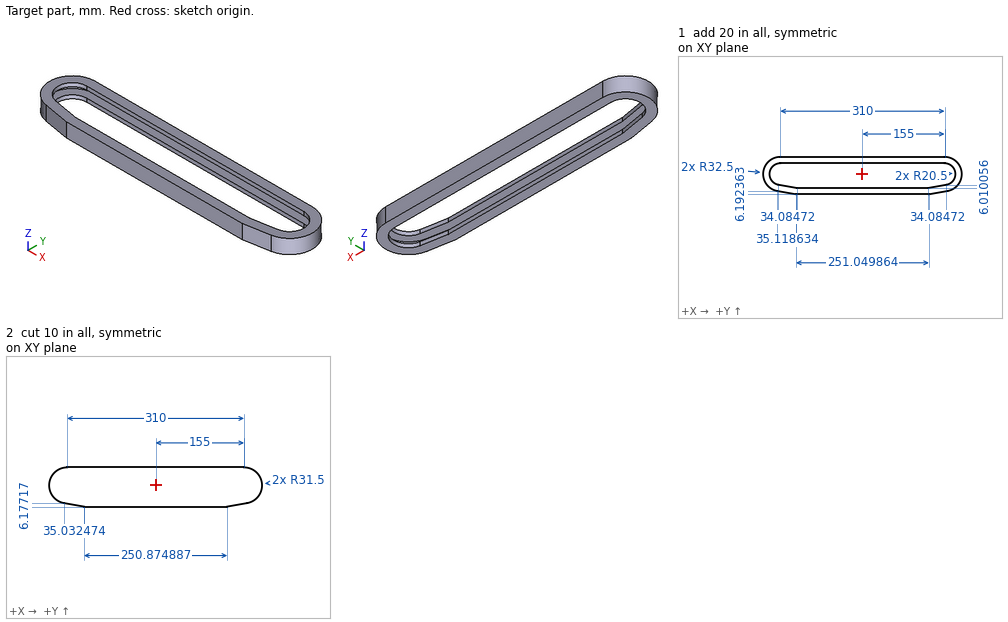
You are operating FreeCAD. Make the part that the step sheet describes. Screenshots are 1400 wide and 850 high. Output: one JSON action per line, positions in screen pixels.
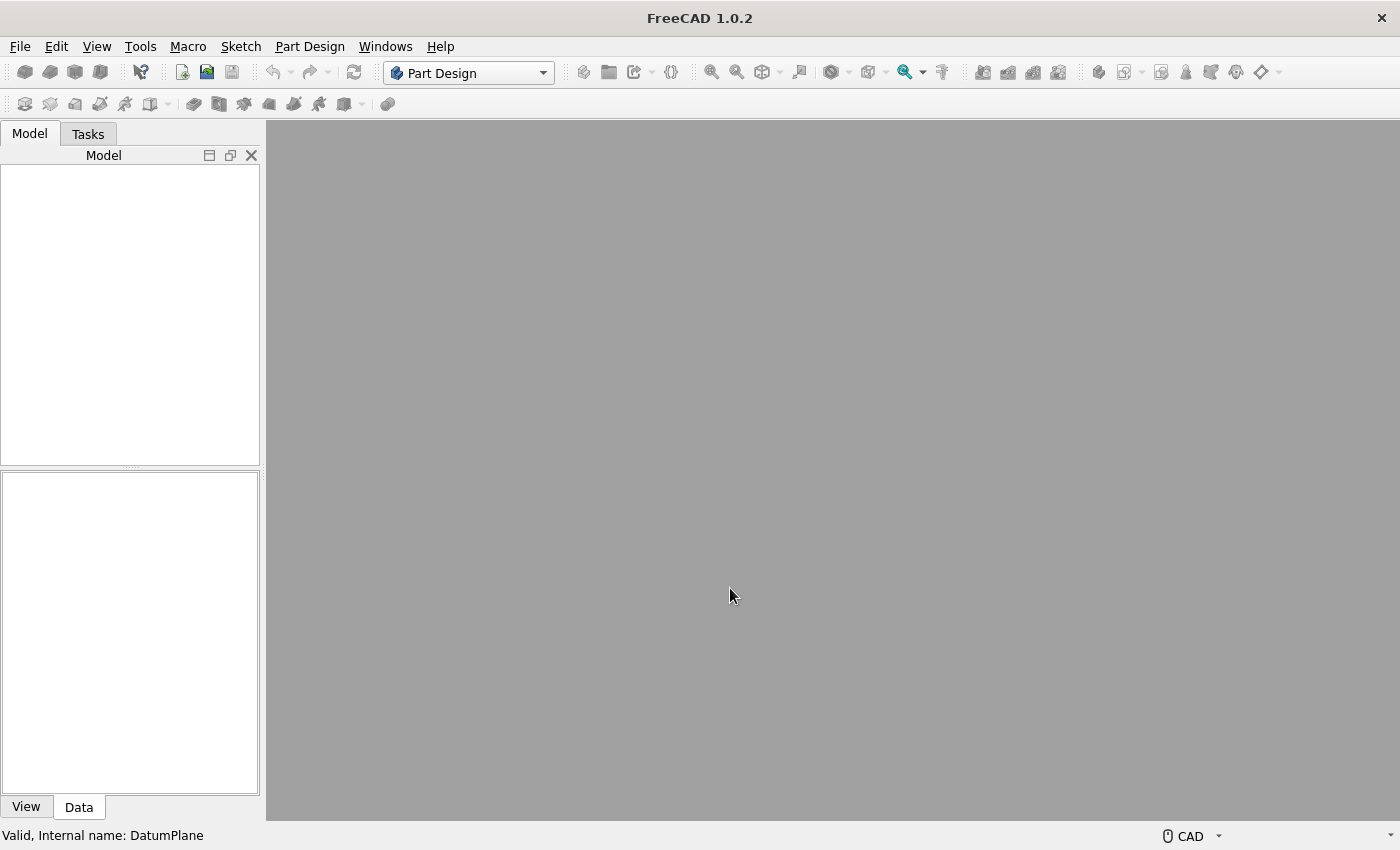
{"action": "left_click", "coordinate": [182, 72]}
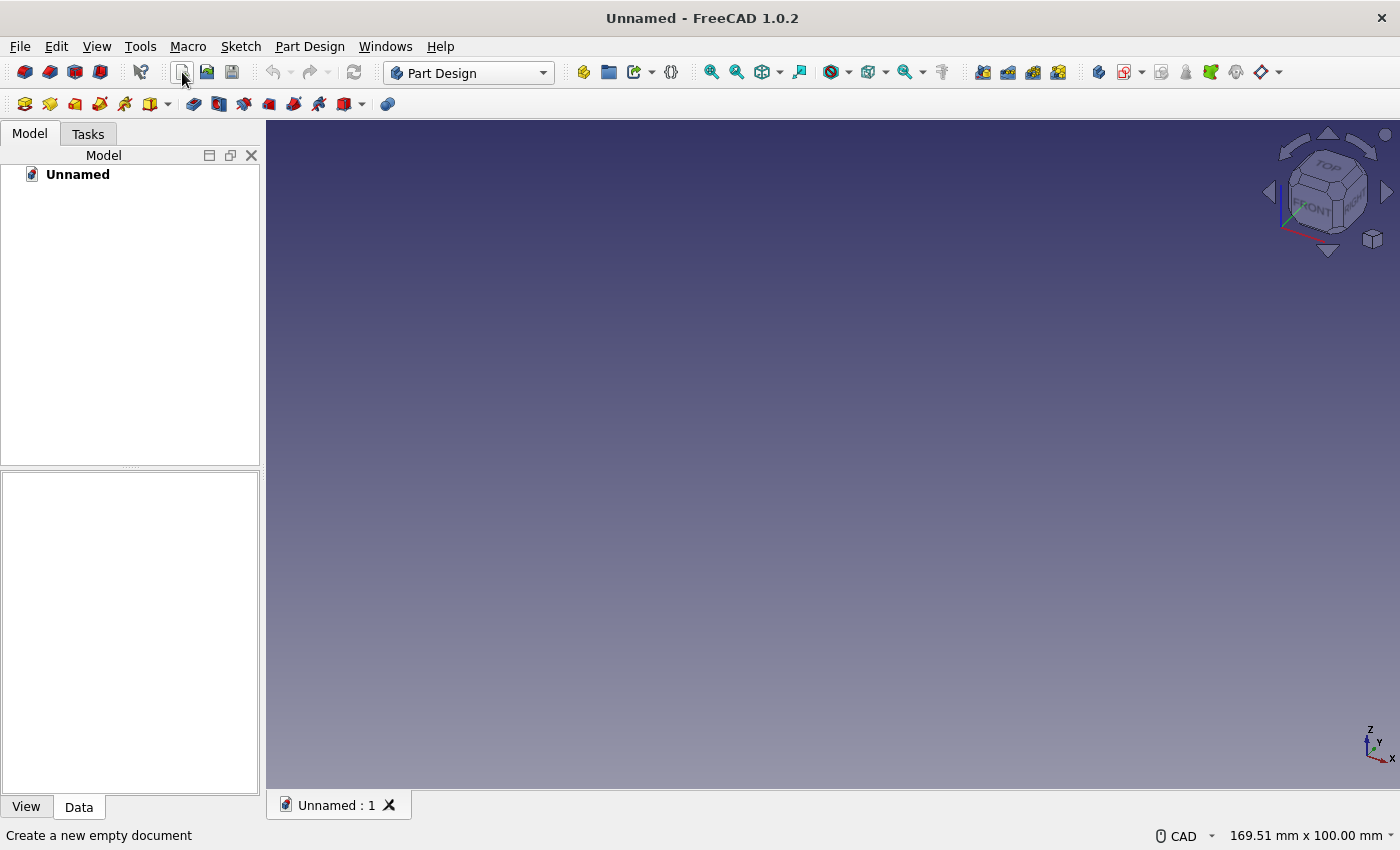
{"action": "left_click", "coordinate": [1124, 72]}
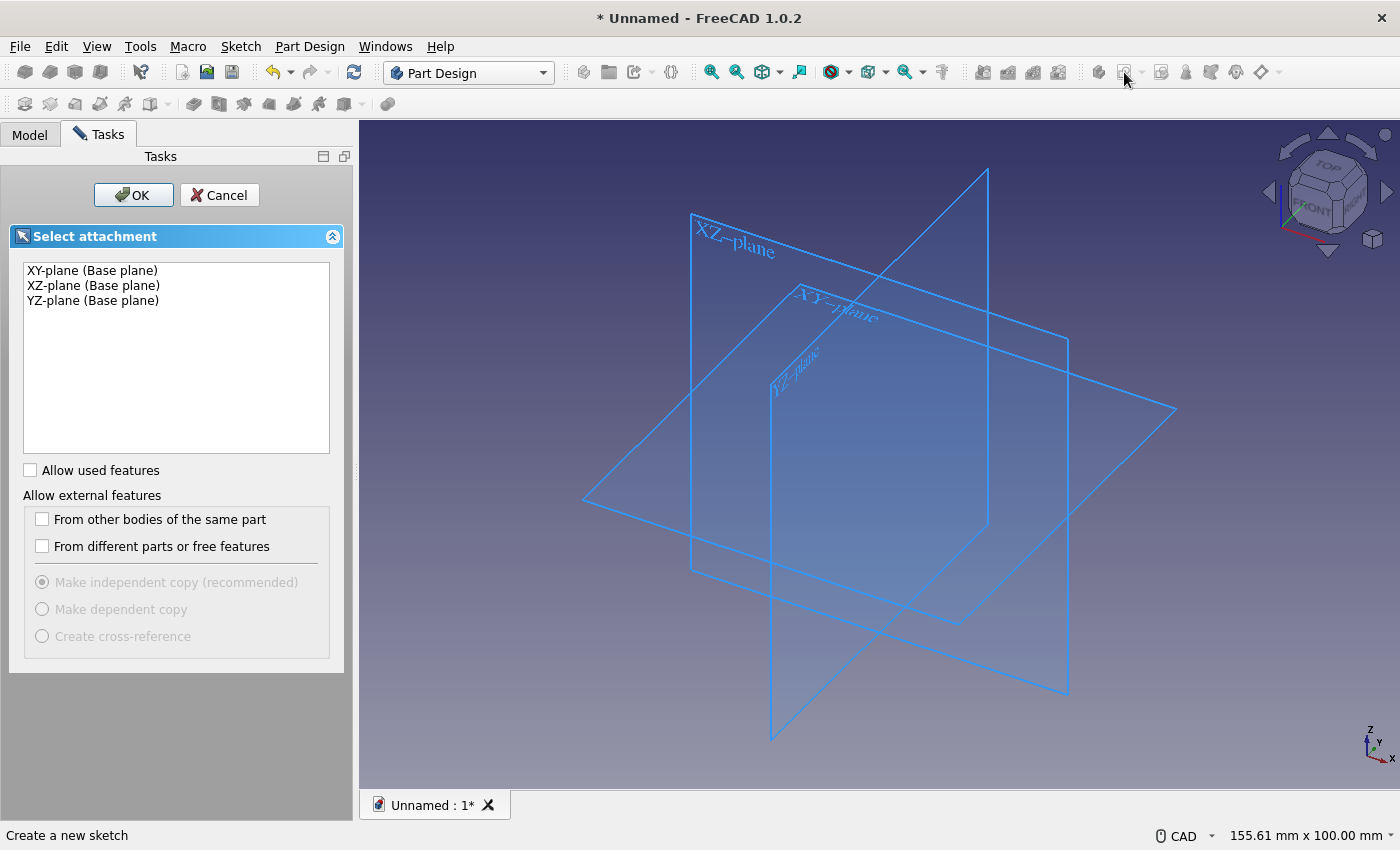
{"action": "left_click", "coordinate": [84, 270]}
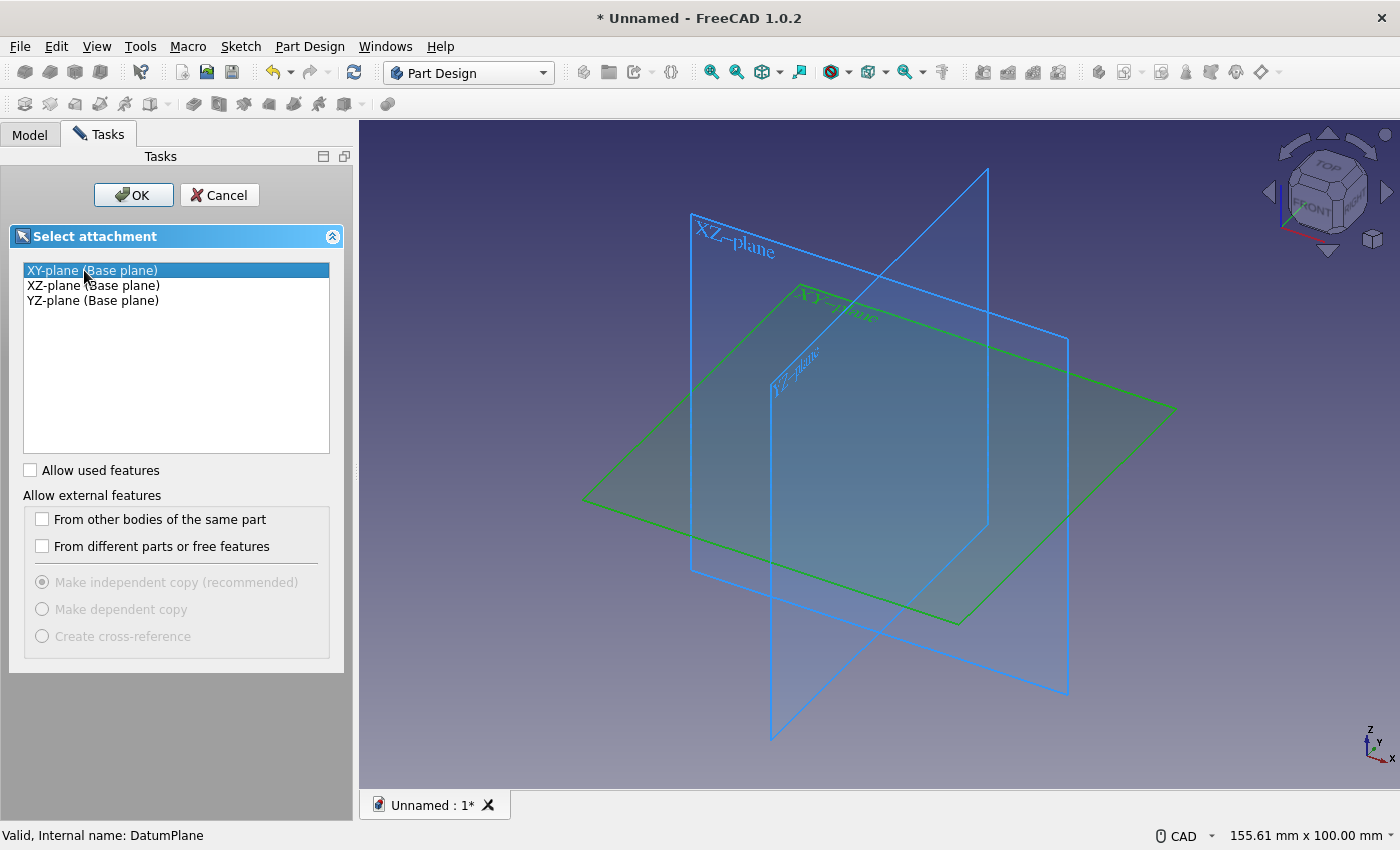
{"action": "left_click", "coordinate": [134, 195]}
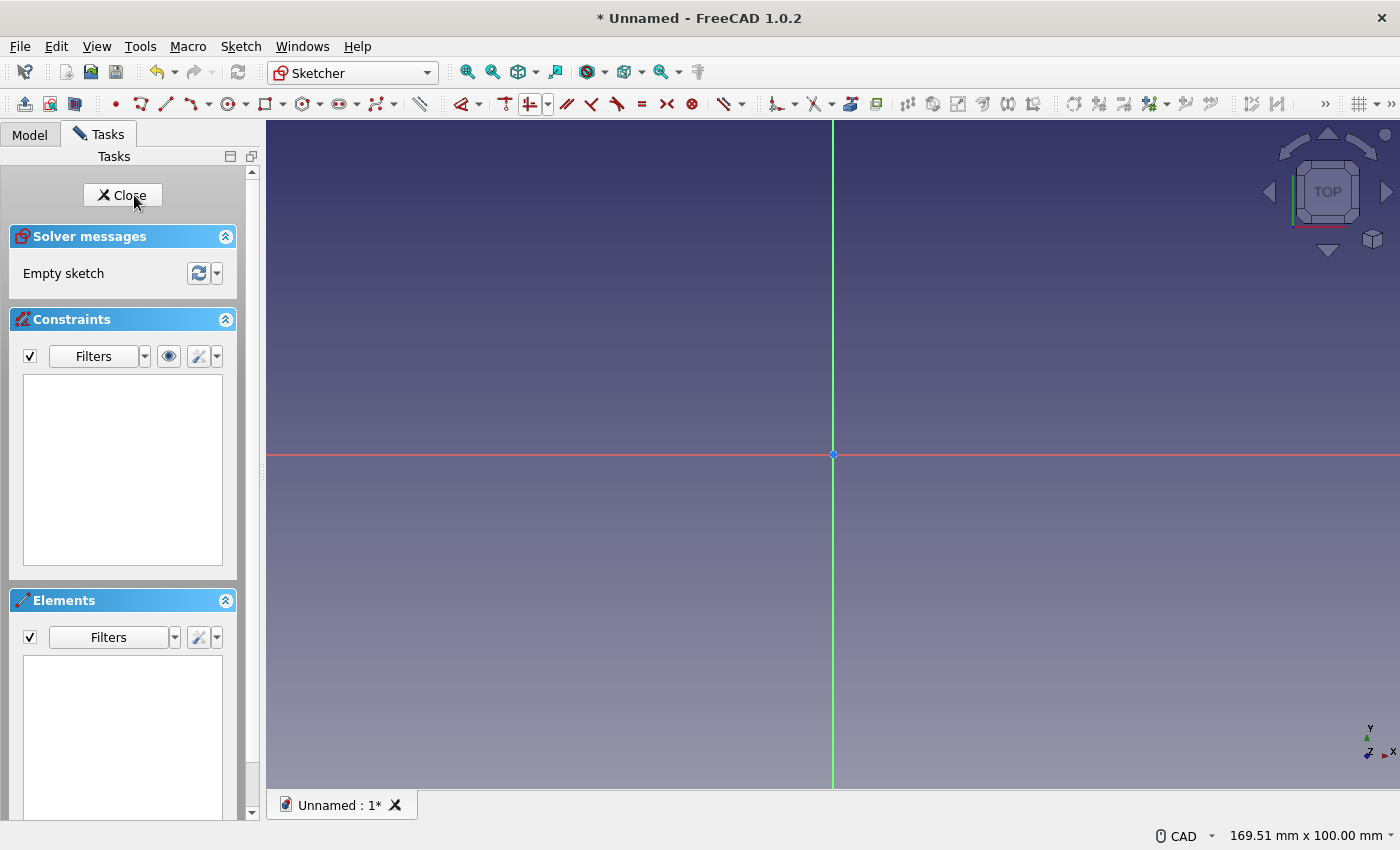
{"action": "scroll", "coordinate": [742, 448], "scroll_direction": "down", "scroll_amount": 7}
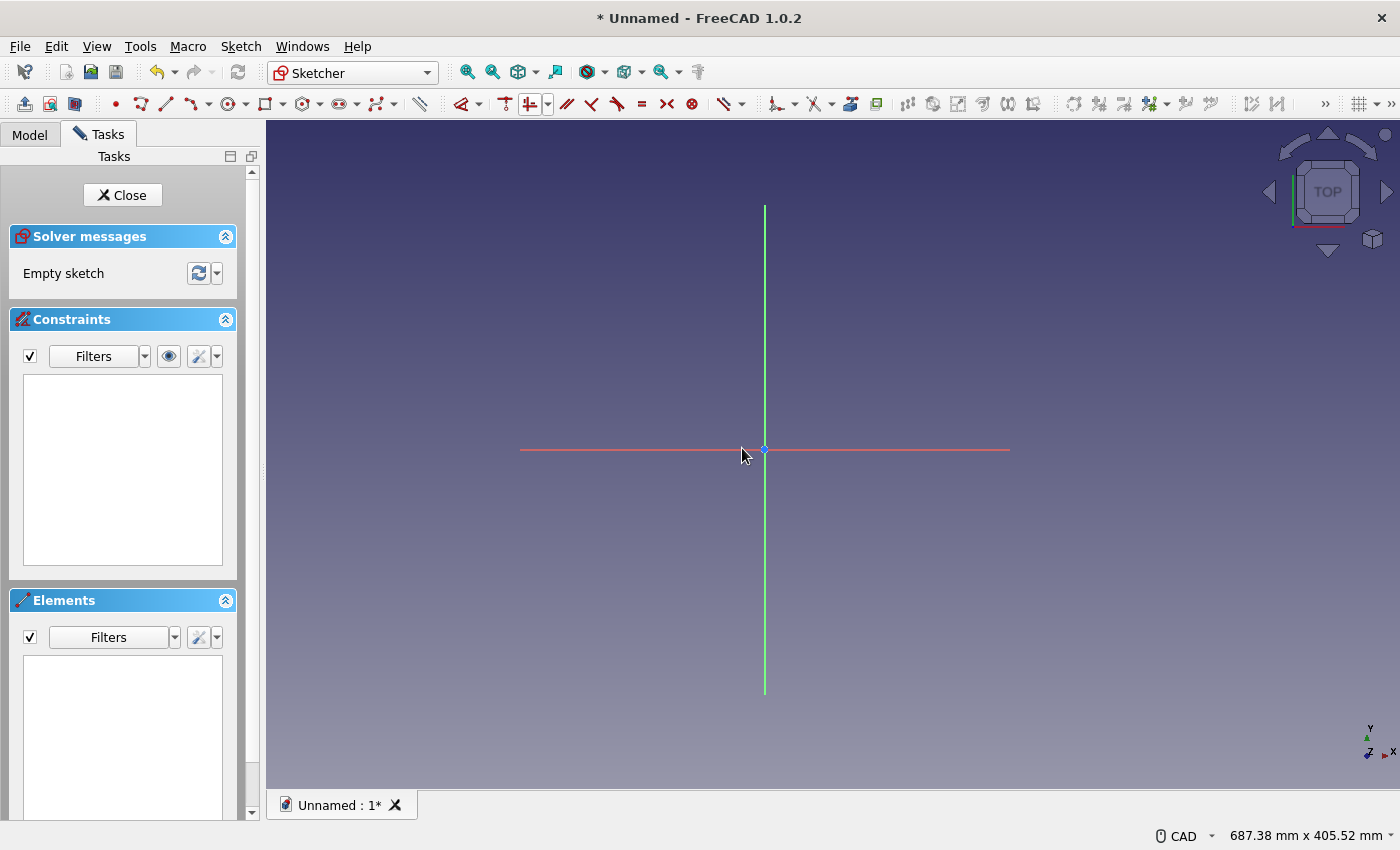
{"action": "left_click", "coordinate": [166, 104]}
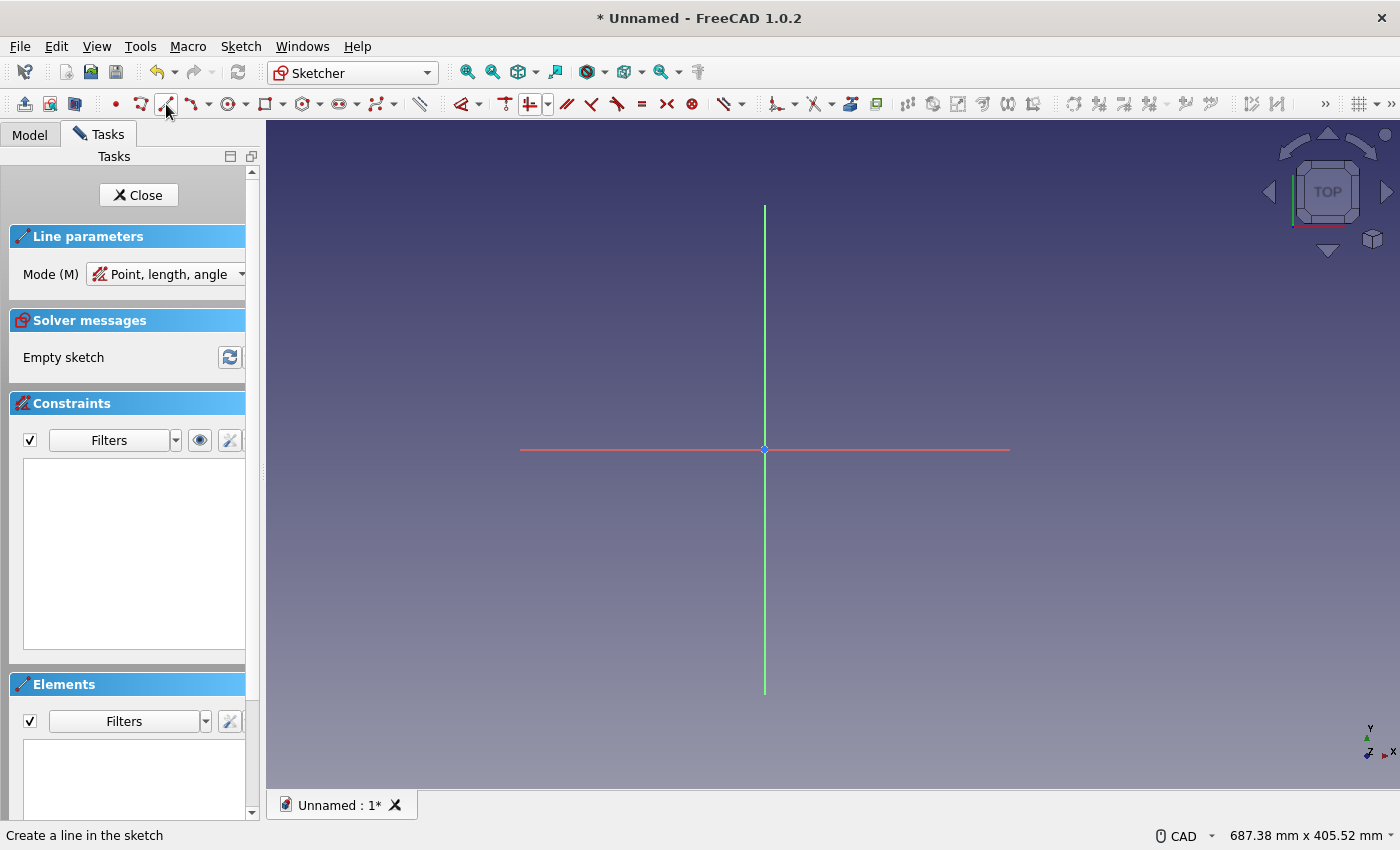
{"action": "left_click", "coordinate": [1020, 396]}
{"action": "left_click", "coordinate": [509, 396]}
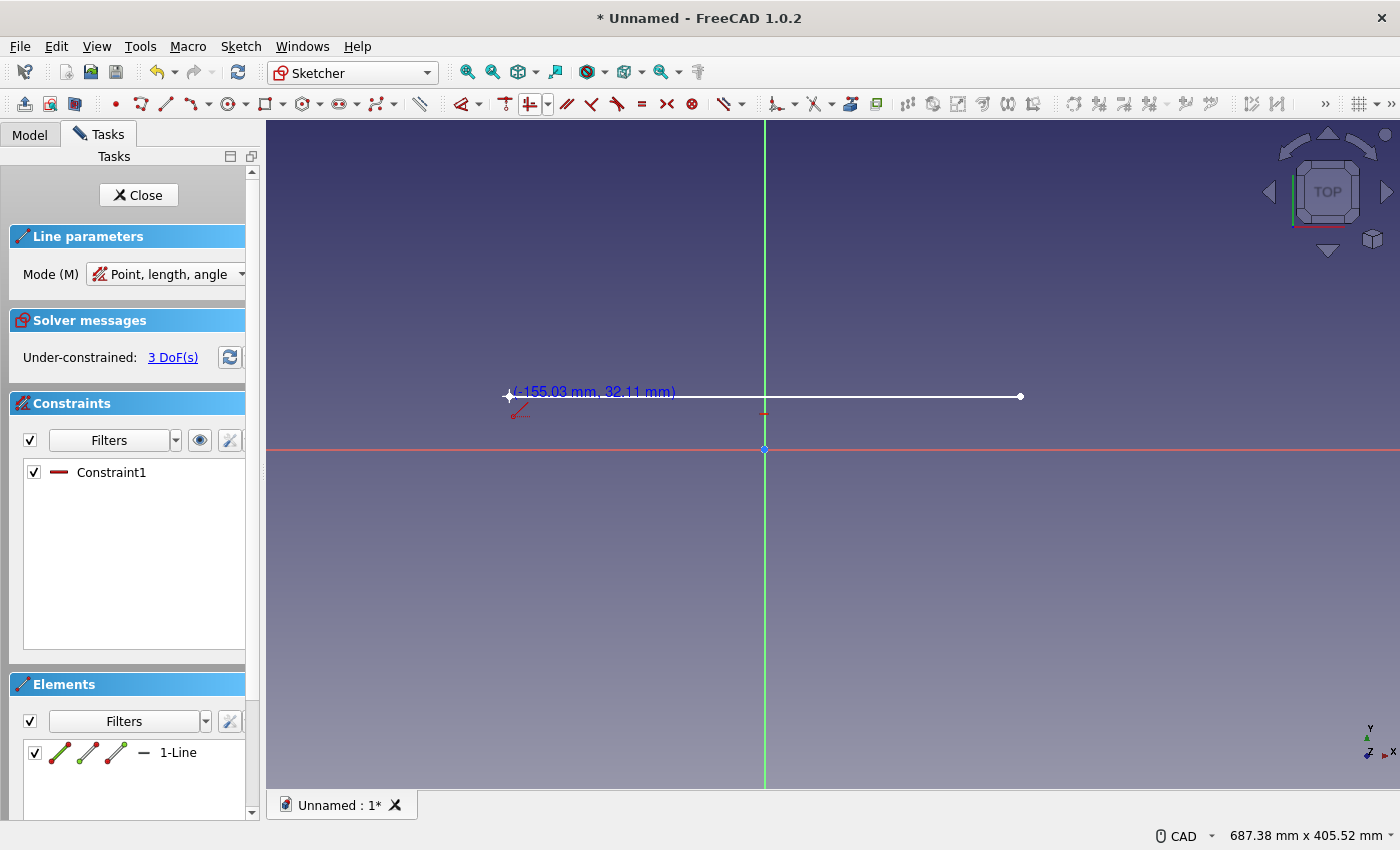
{"action": "left_click", "coordinate": [141, 104]}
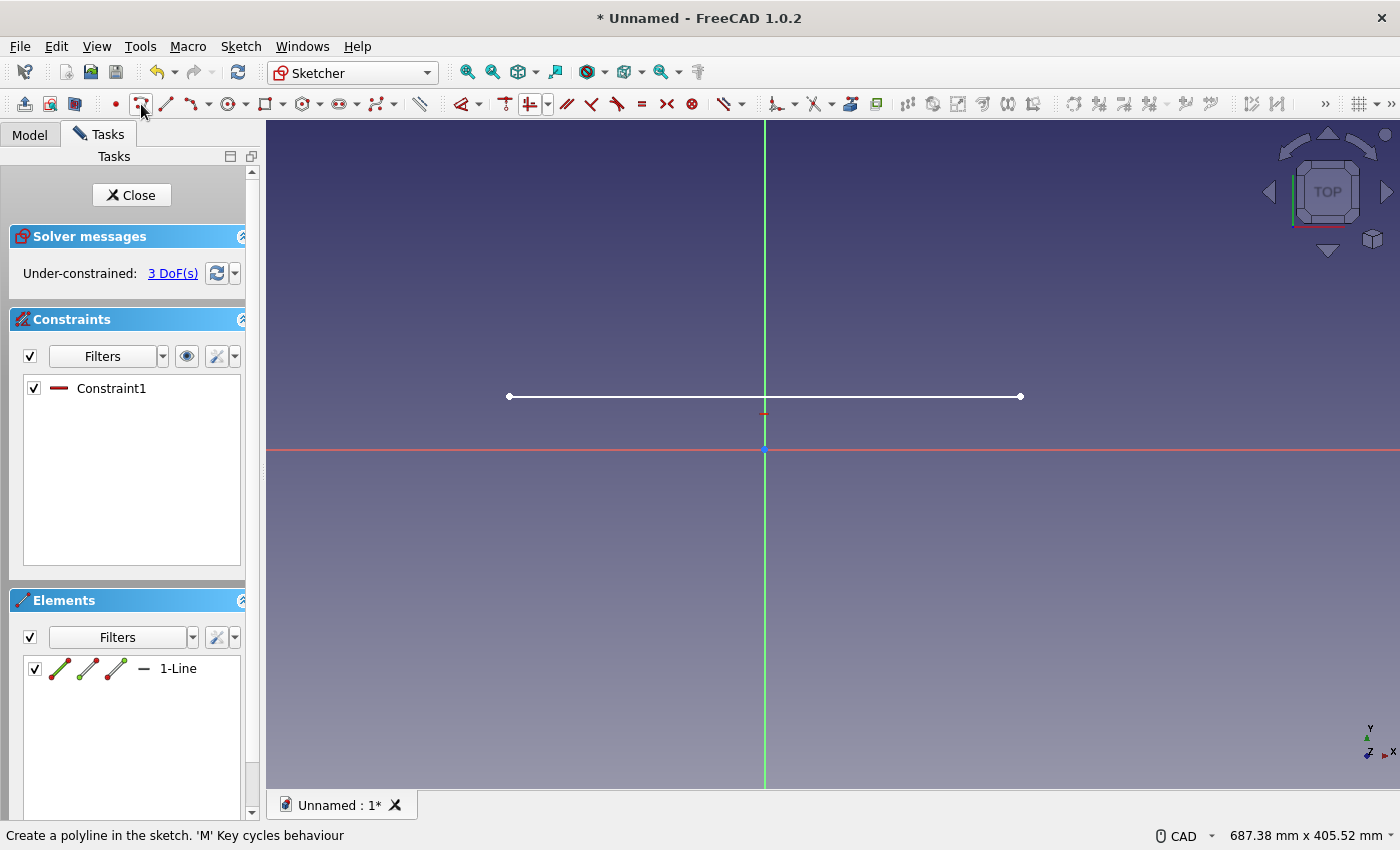
{"action": "left_click", "coordinate": [500, 503]}
{"action": "left_click", "coordinate": [558, 513]}
{"action": "left_click", "coordinate": [972, 513]}
{"action": "left_click", "coordinate": [1030, 503]}
{"action": "right_click", "coordinate": [1030, 503]}